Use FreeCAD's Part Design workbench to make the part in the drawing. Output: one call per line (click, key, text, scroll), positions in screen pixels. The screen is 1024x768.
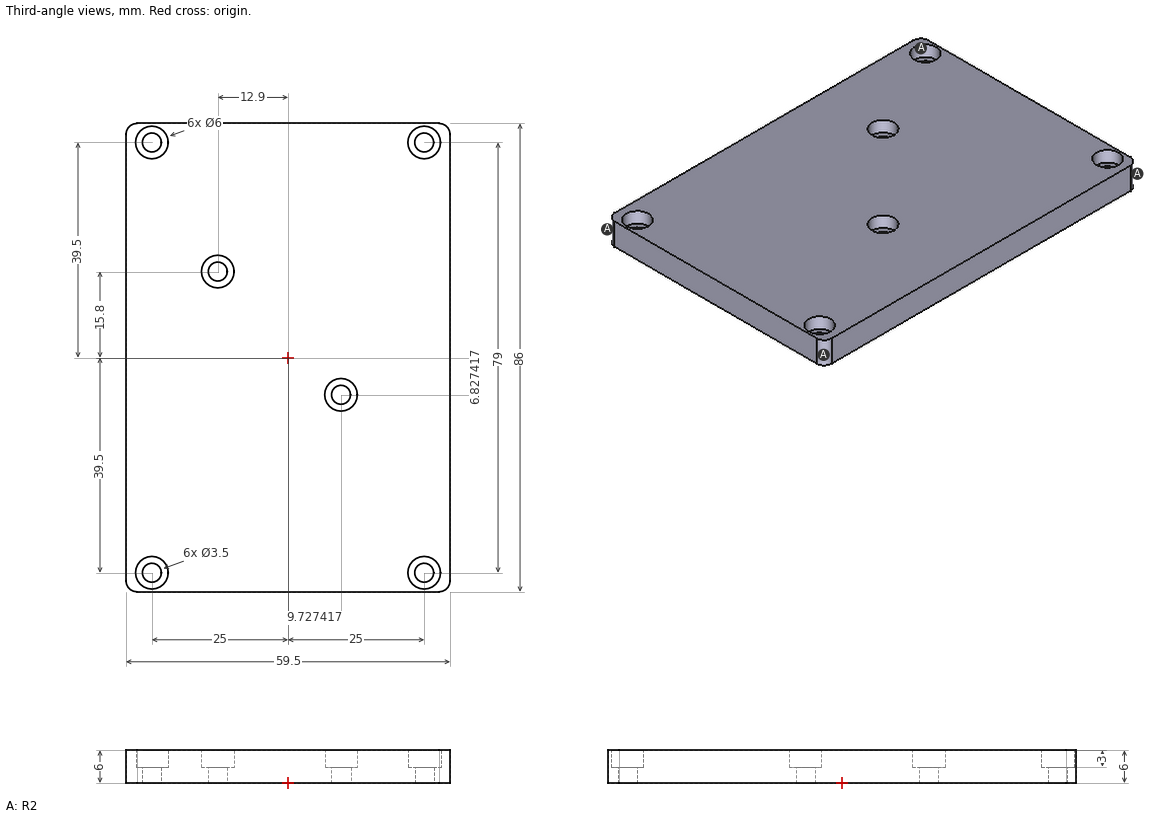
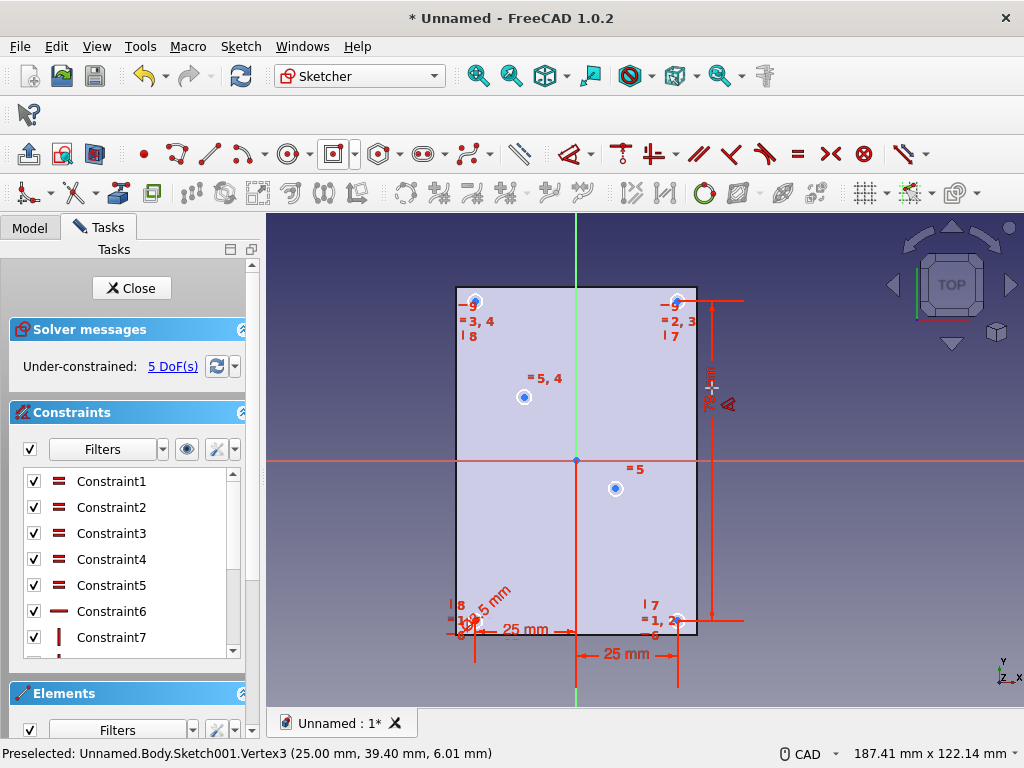
click(475, 621)
click(441, 541)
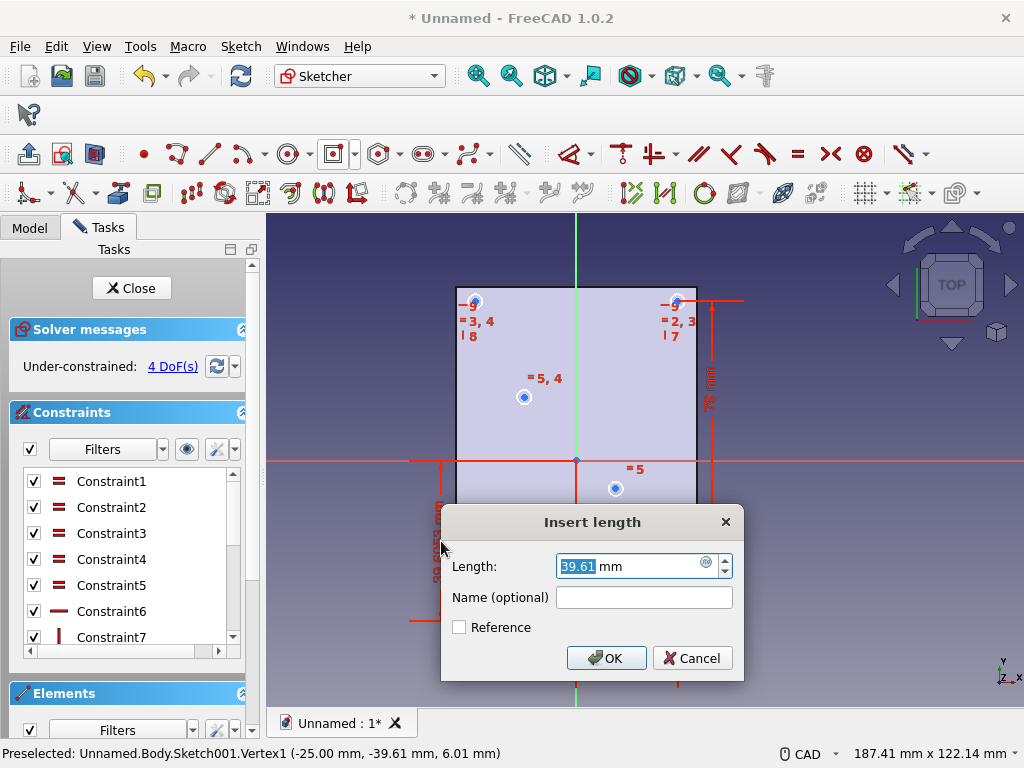
text(39.5)
key(Return)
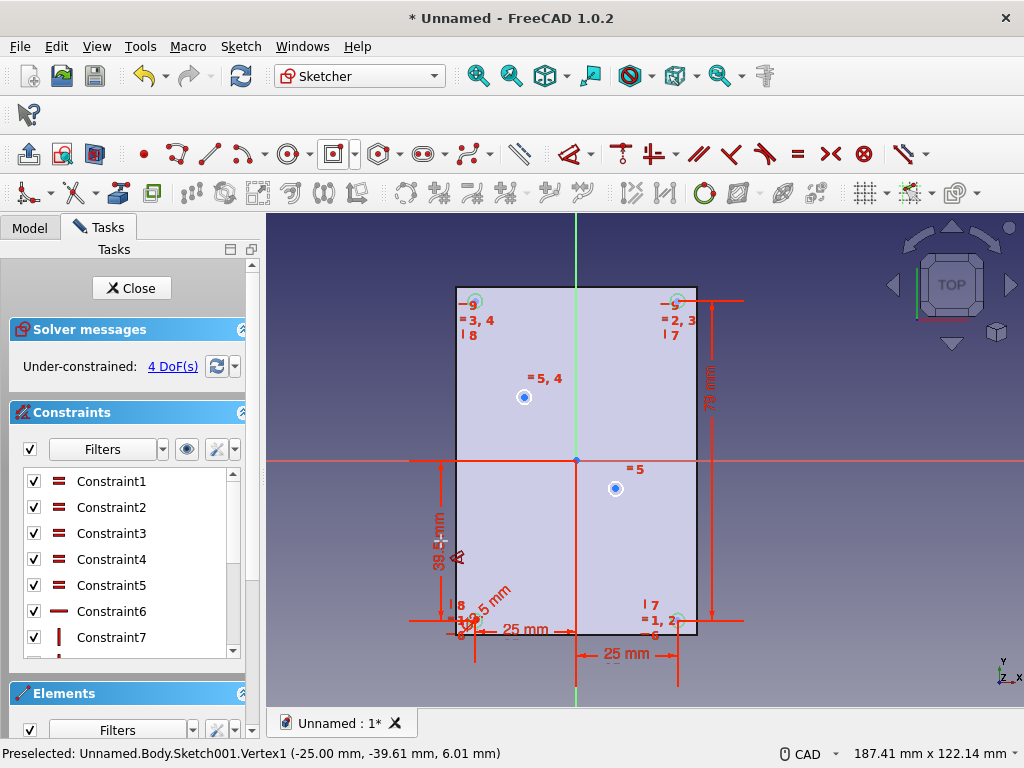
click(524, 397)
click(550, 363)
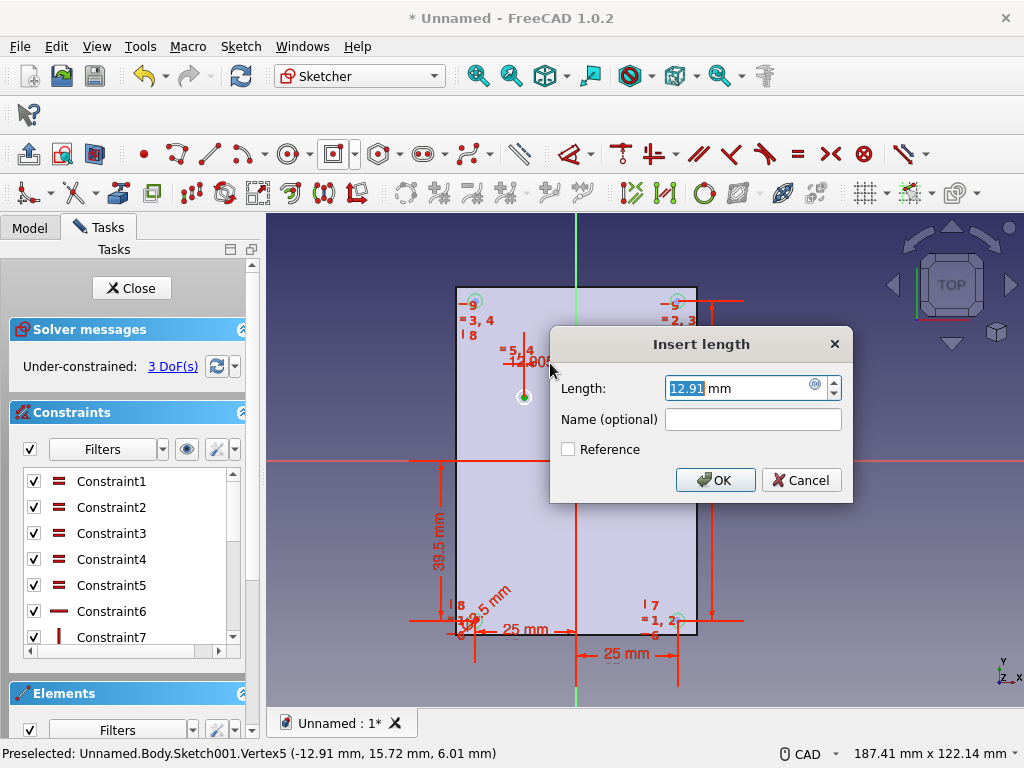
text(12.9)
key(Return)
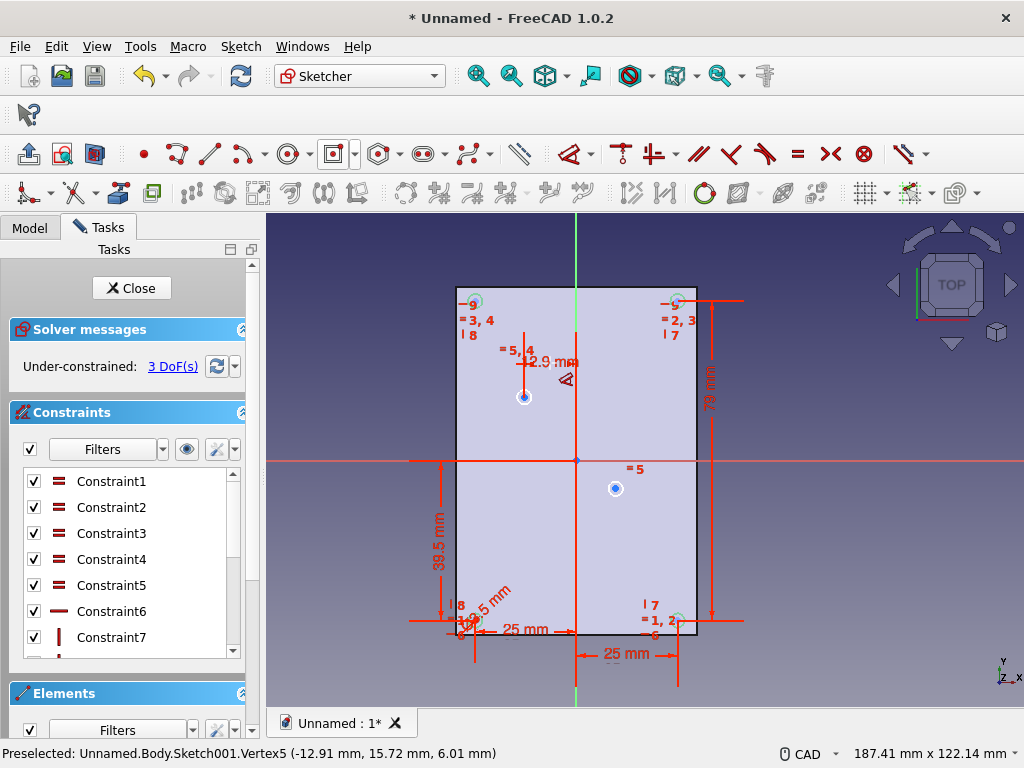
click(524, 397)
click(490, 429)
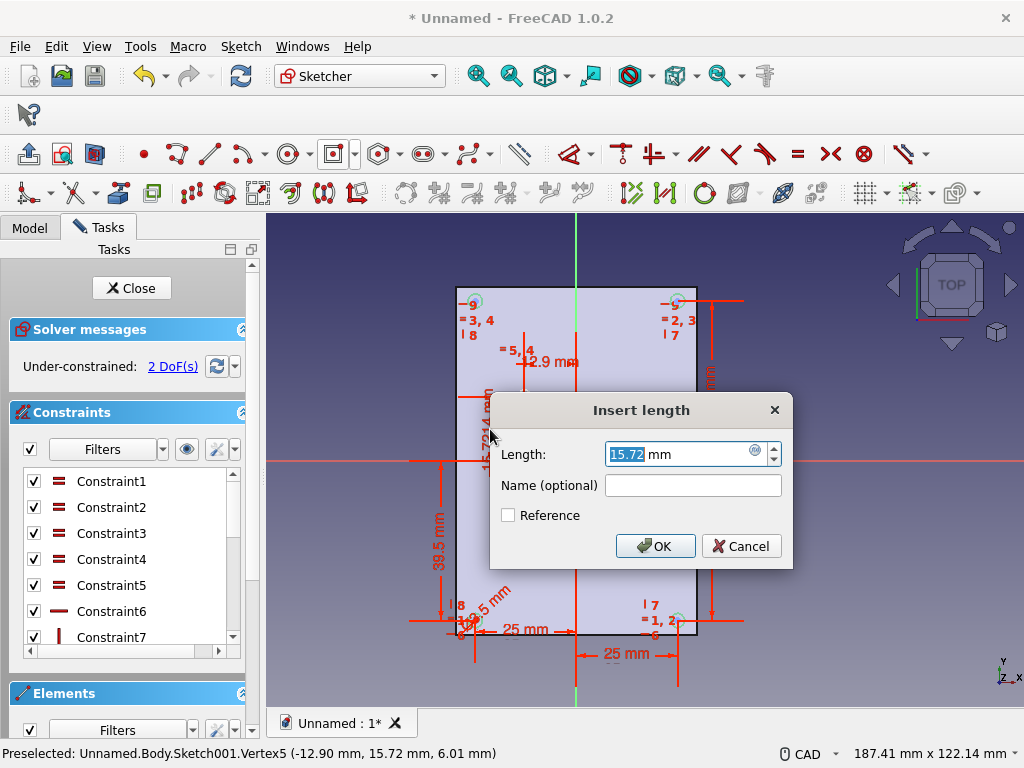
text(15.8)
key(Return)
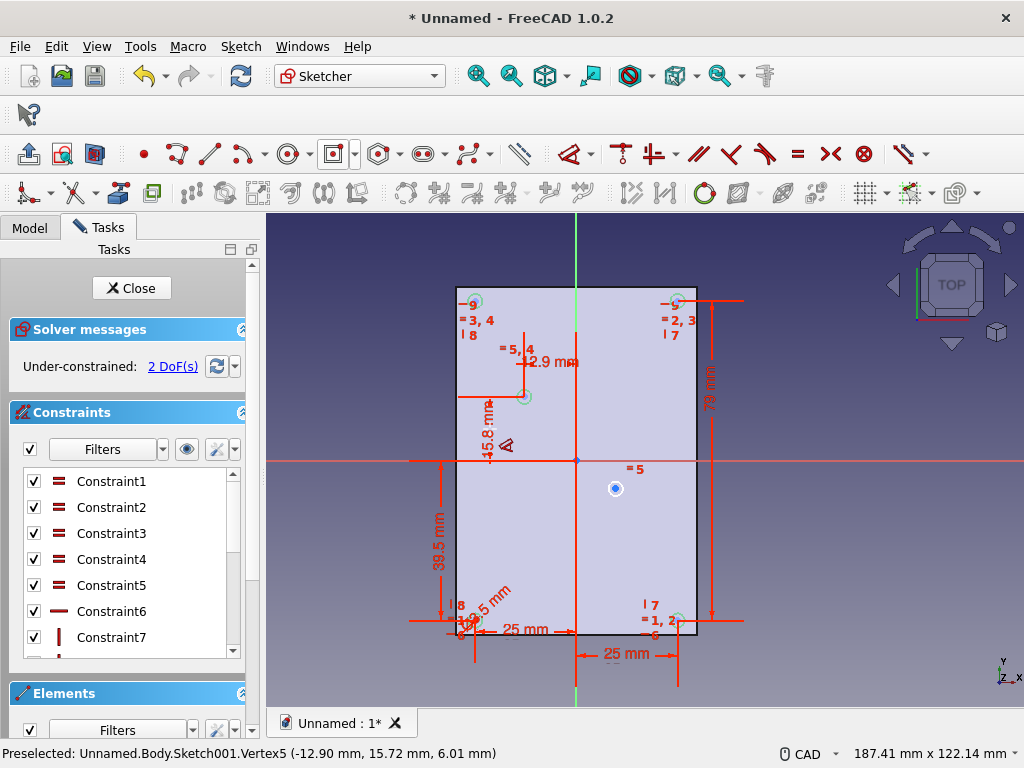
click(616, 489)
click(596, 523)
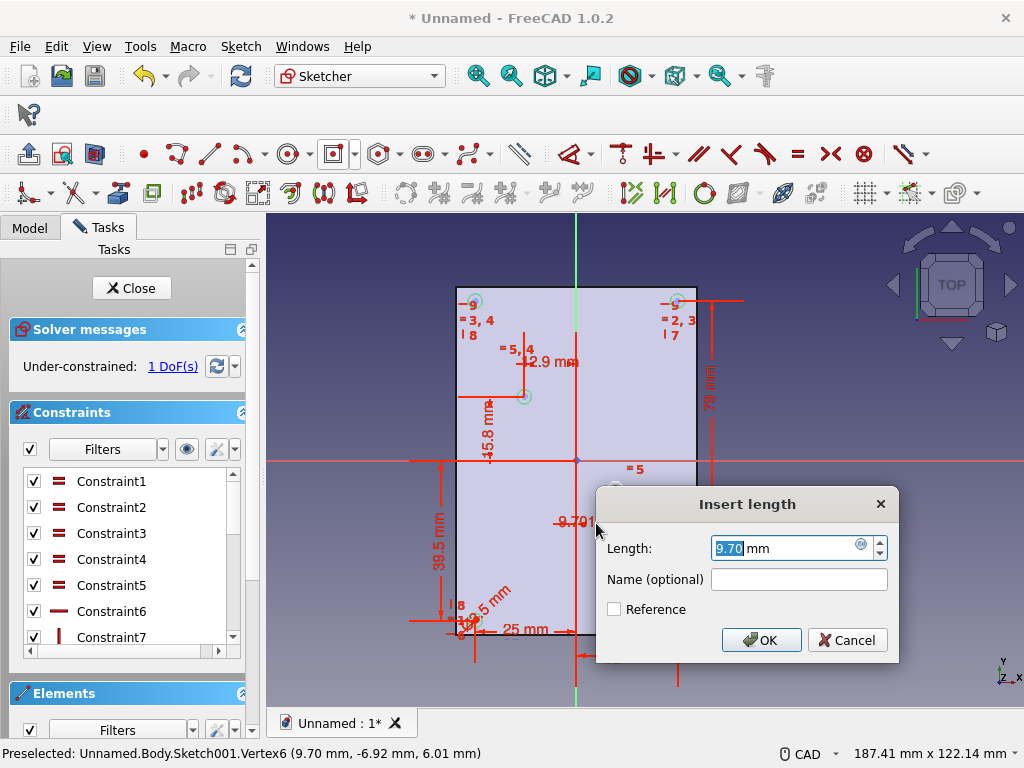
text(9.727417)
key(Return)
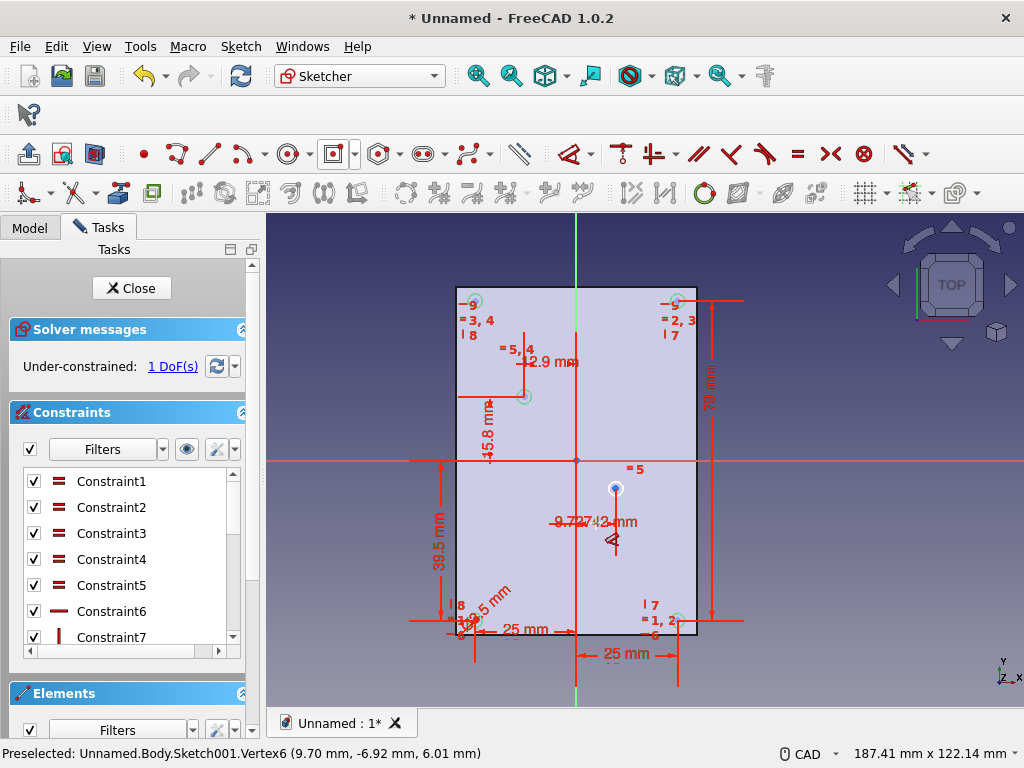
scroll(616, 489, up, 2)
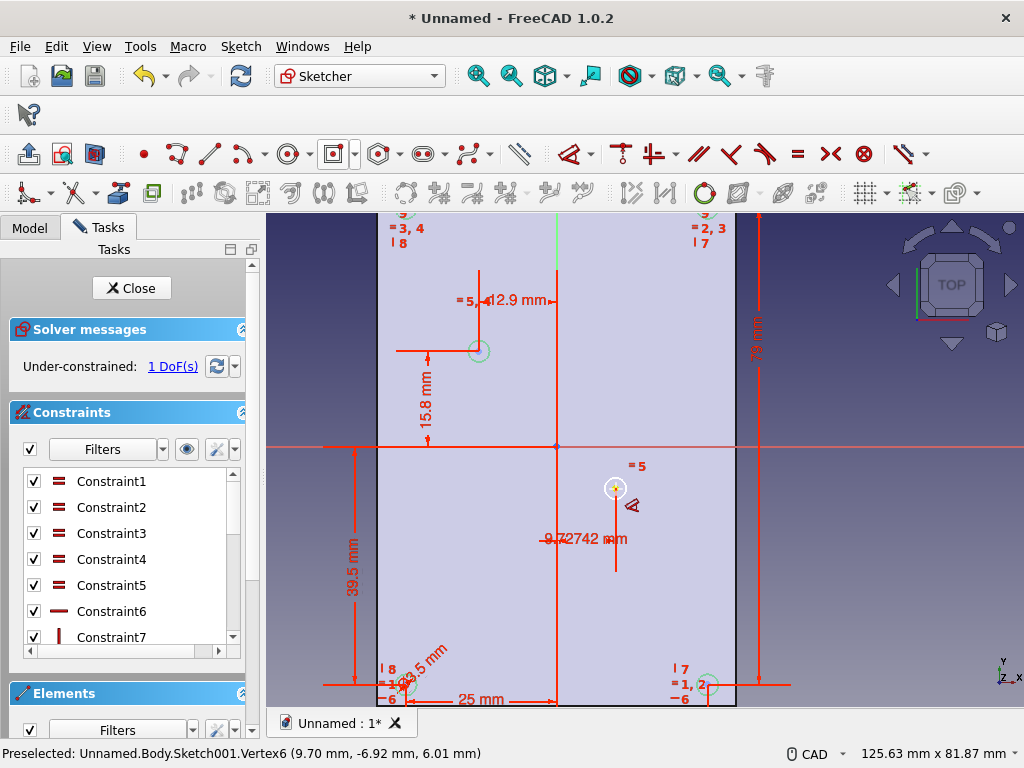
click(616, 488)
click(650, 468)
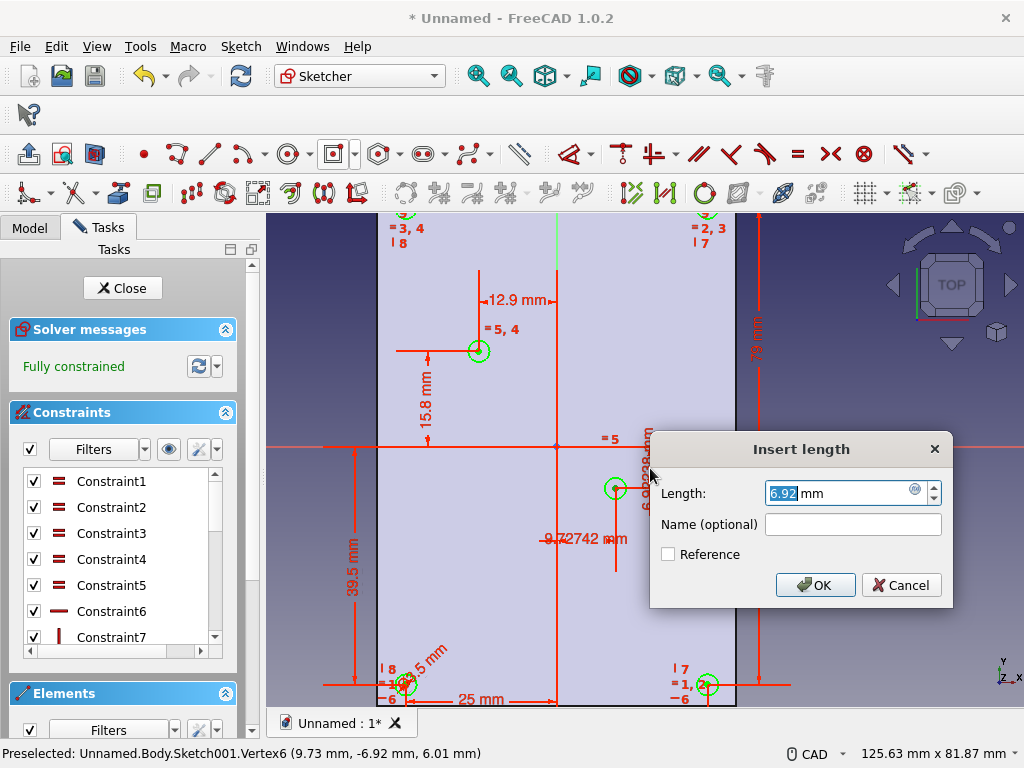
text(6.827417)
key(Return)
key(Escape)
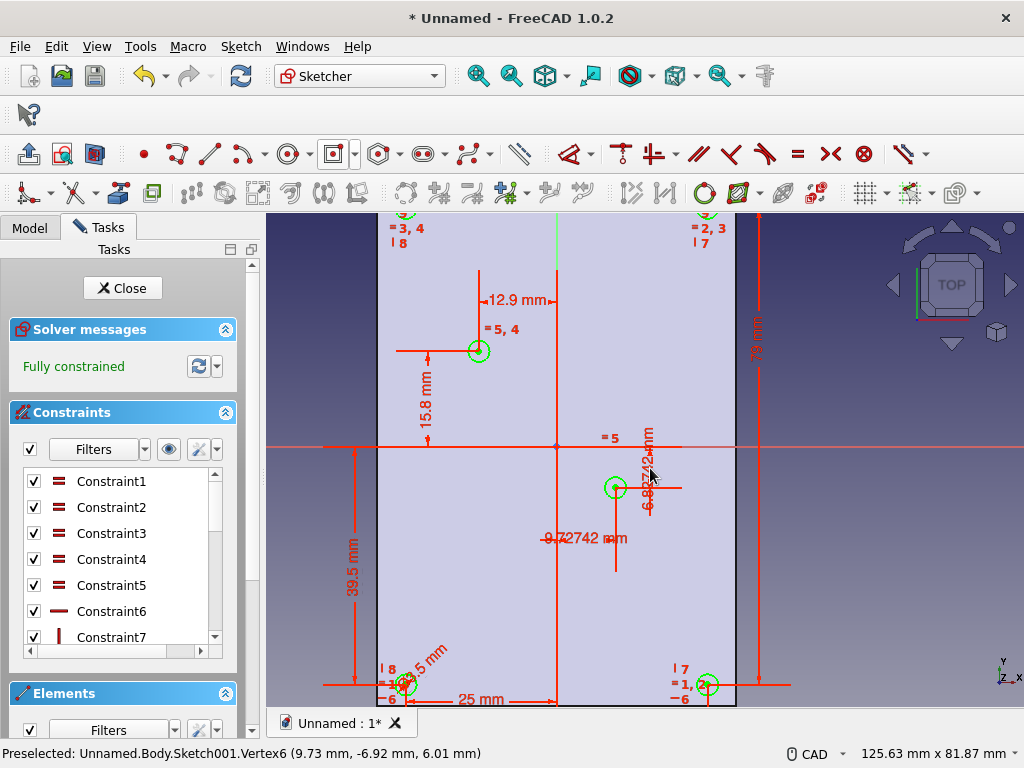
click(123, 288)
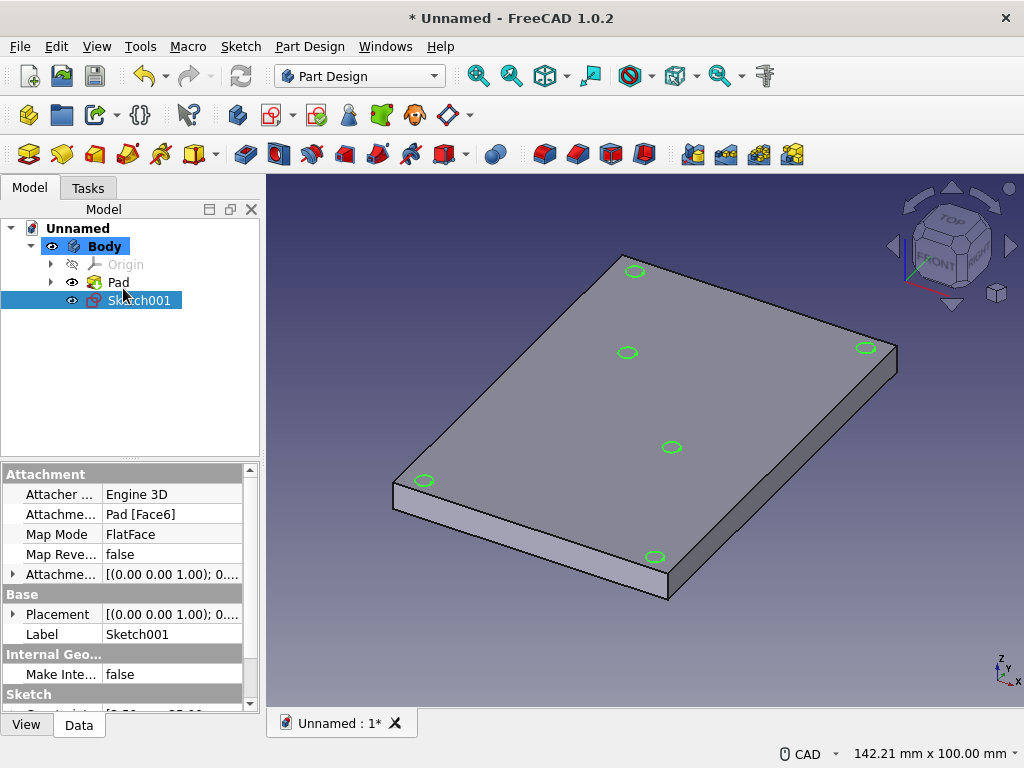
click(246, 154)